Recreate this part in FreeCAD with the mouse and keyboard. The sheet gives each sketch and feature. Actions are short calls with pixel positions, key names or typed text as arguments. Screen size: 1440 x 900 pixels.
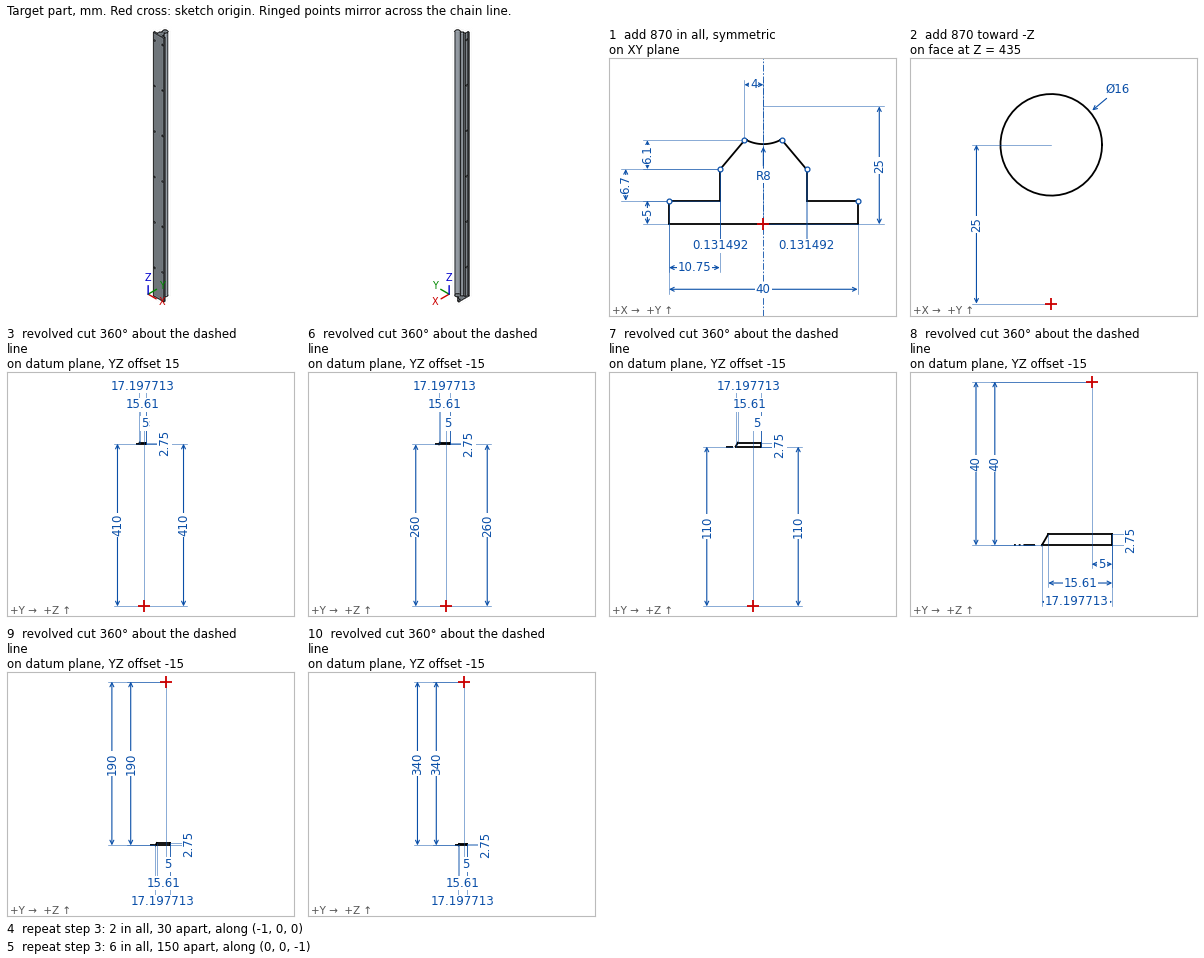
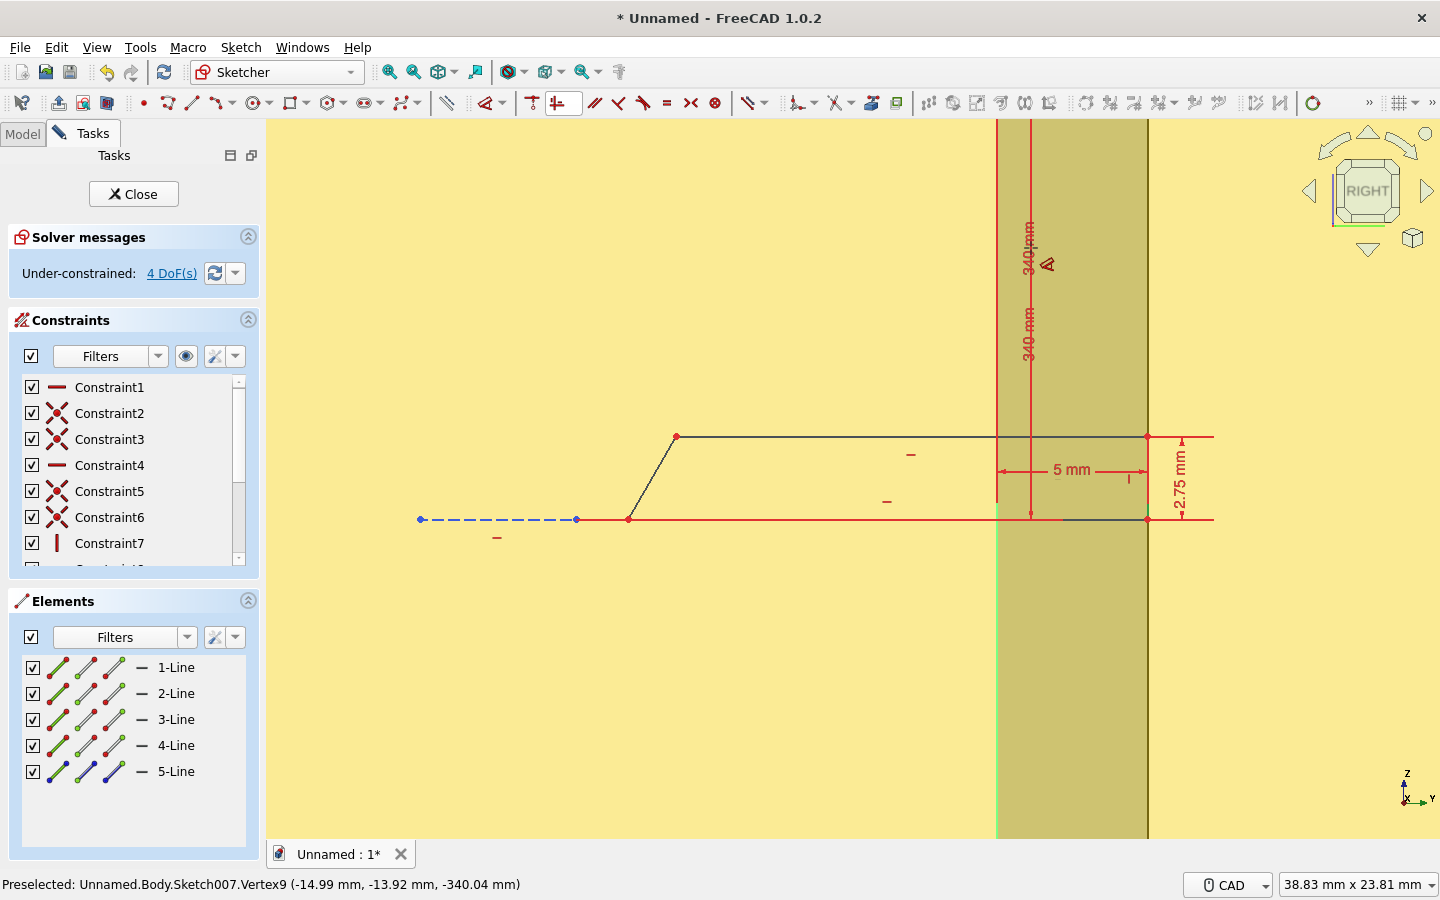
scroll(1006, 437, up, 2)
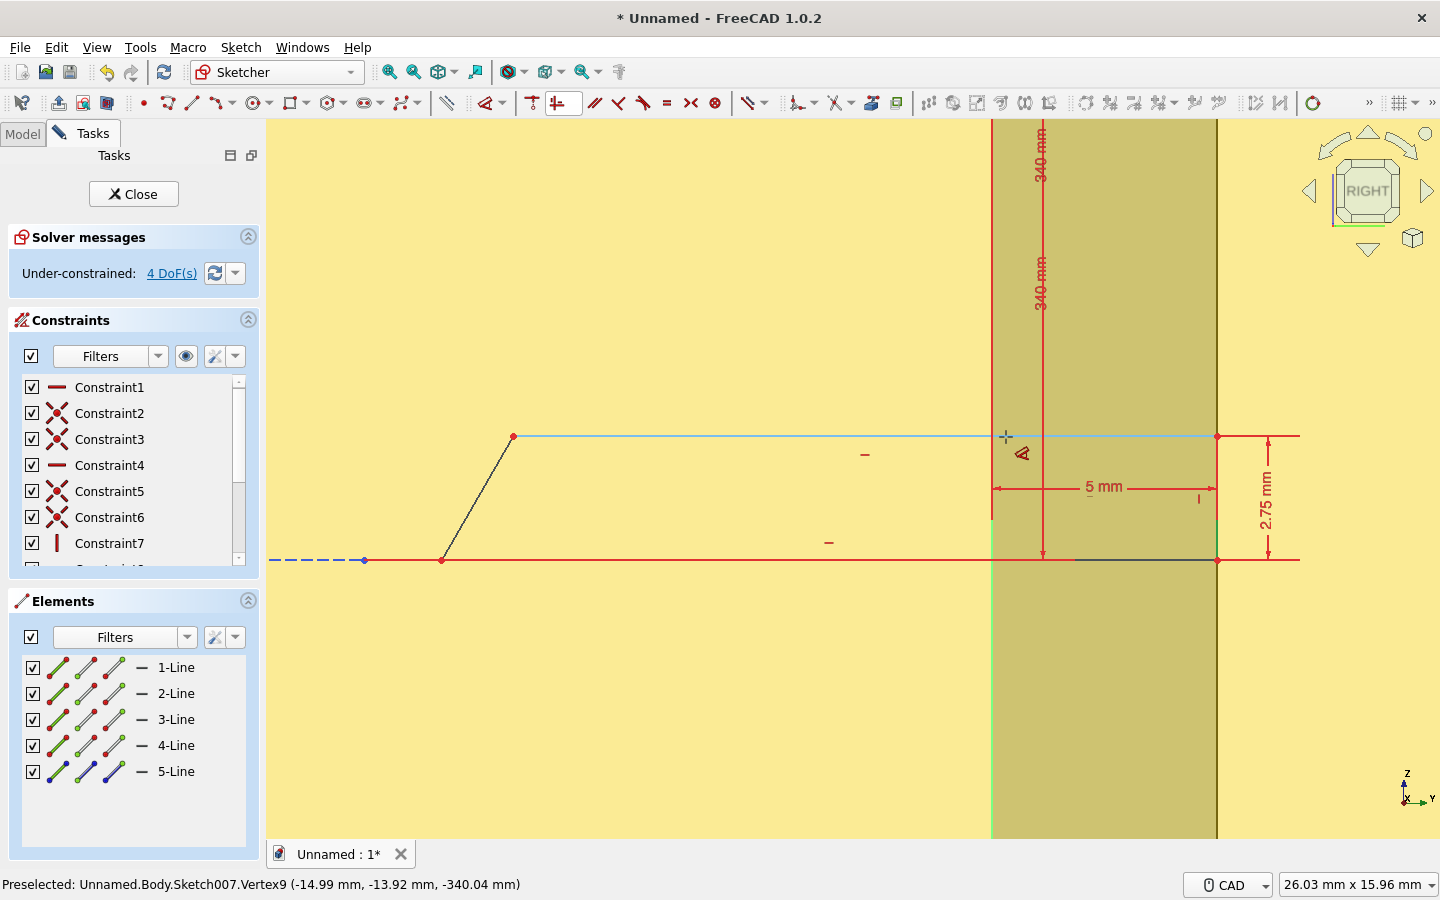
click(1006, 436)
click(865, 402)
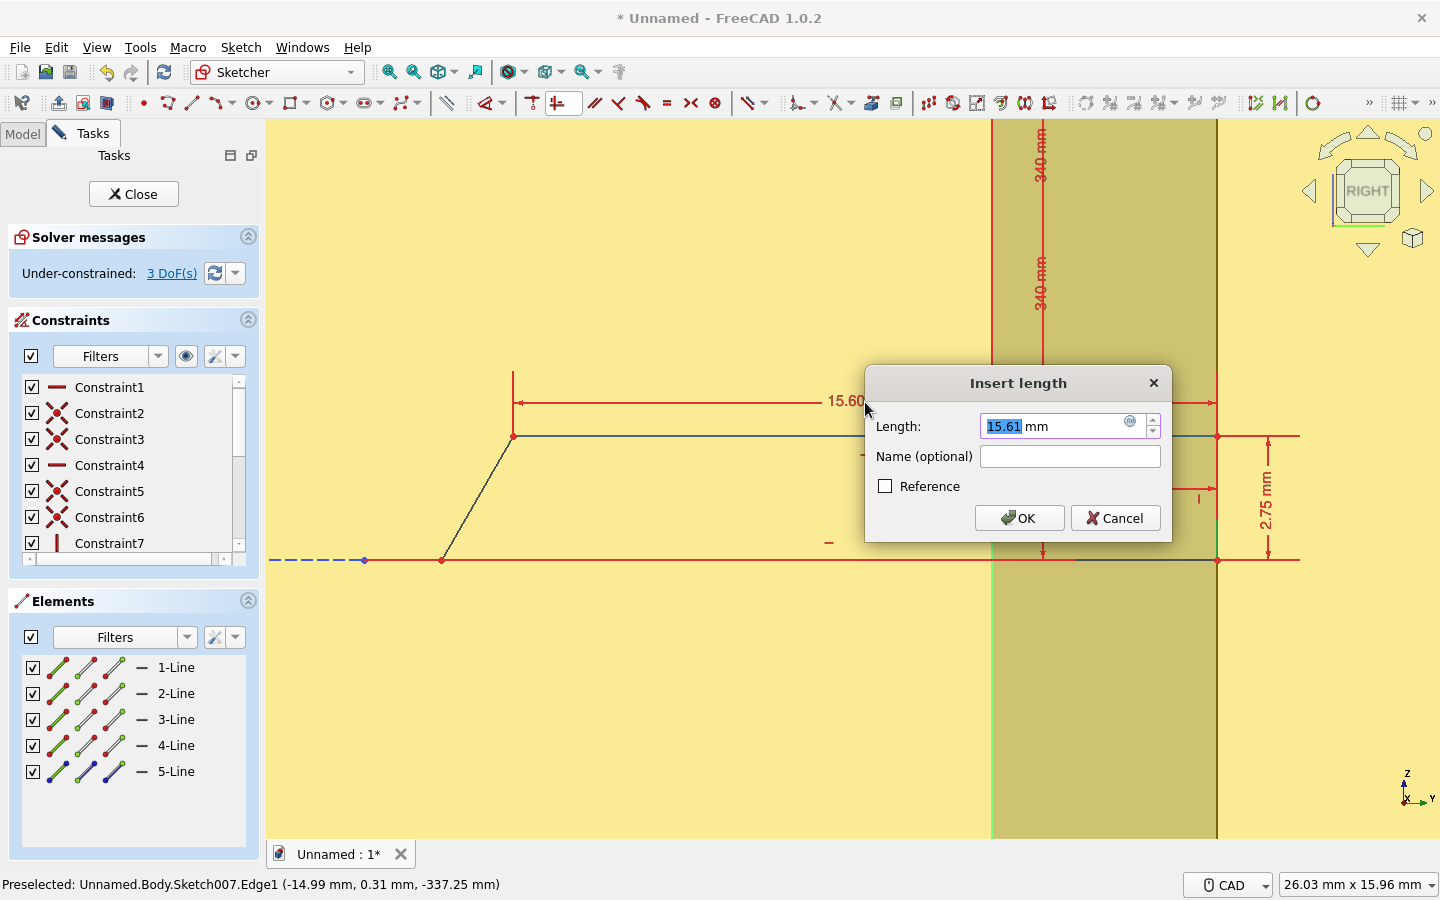
text(15.61)
key(Return)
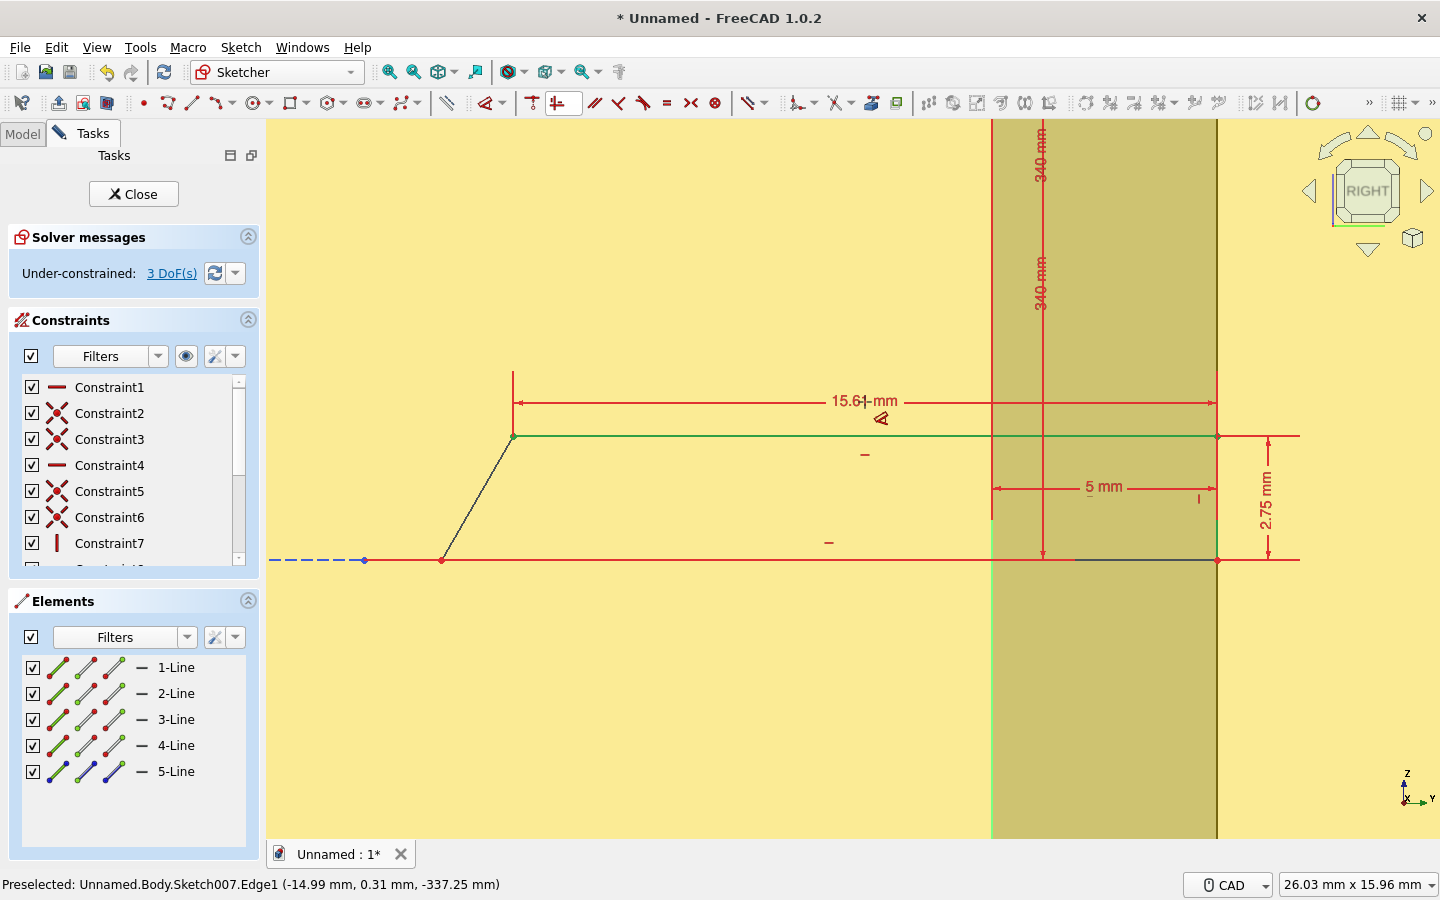
click(674, 560)
click(830, 594)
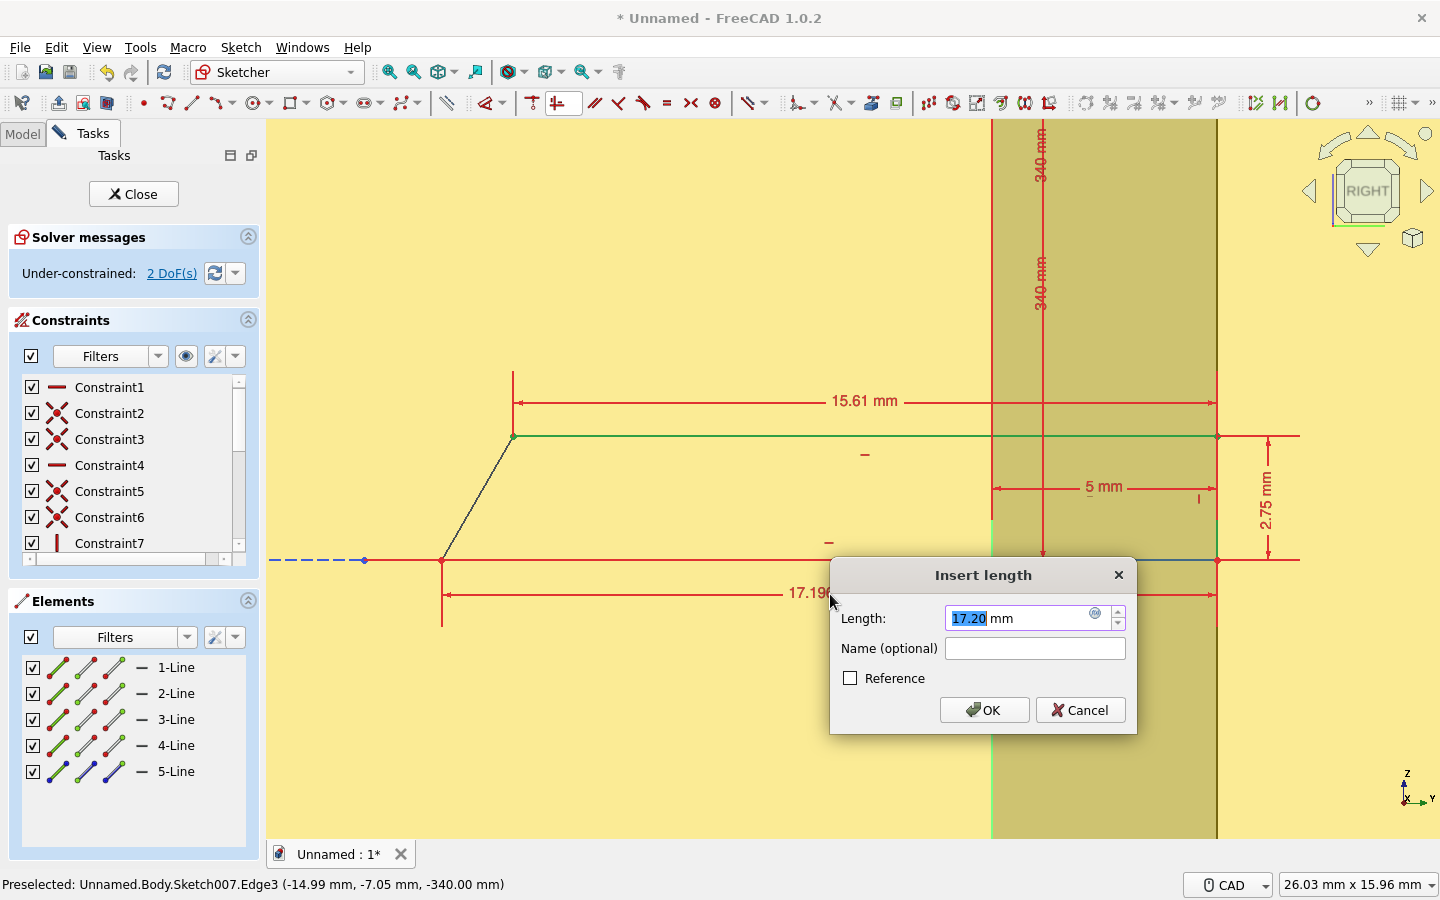
text(17.197713)
key(Return)
key(Escape)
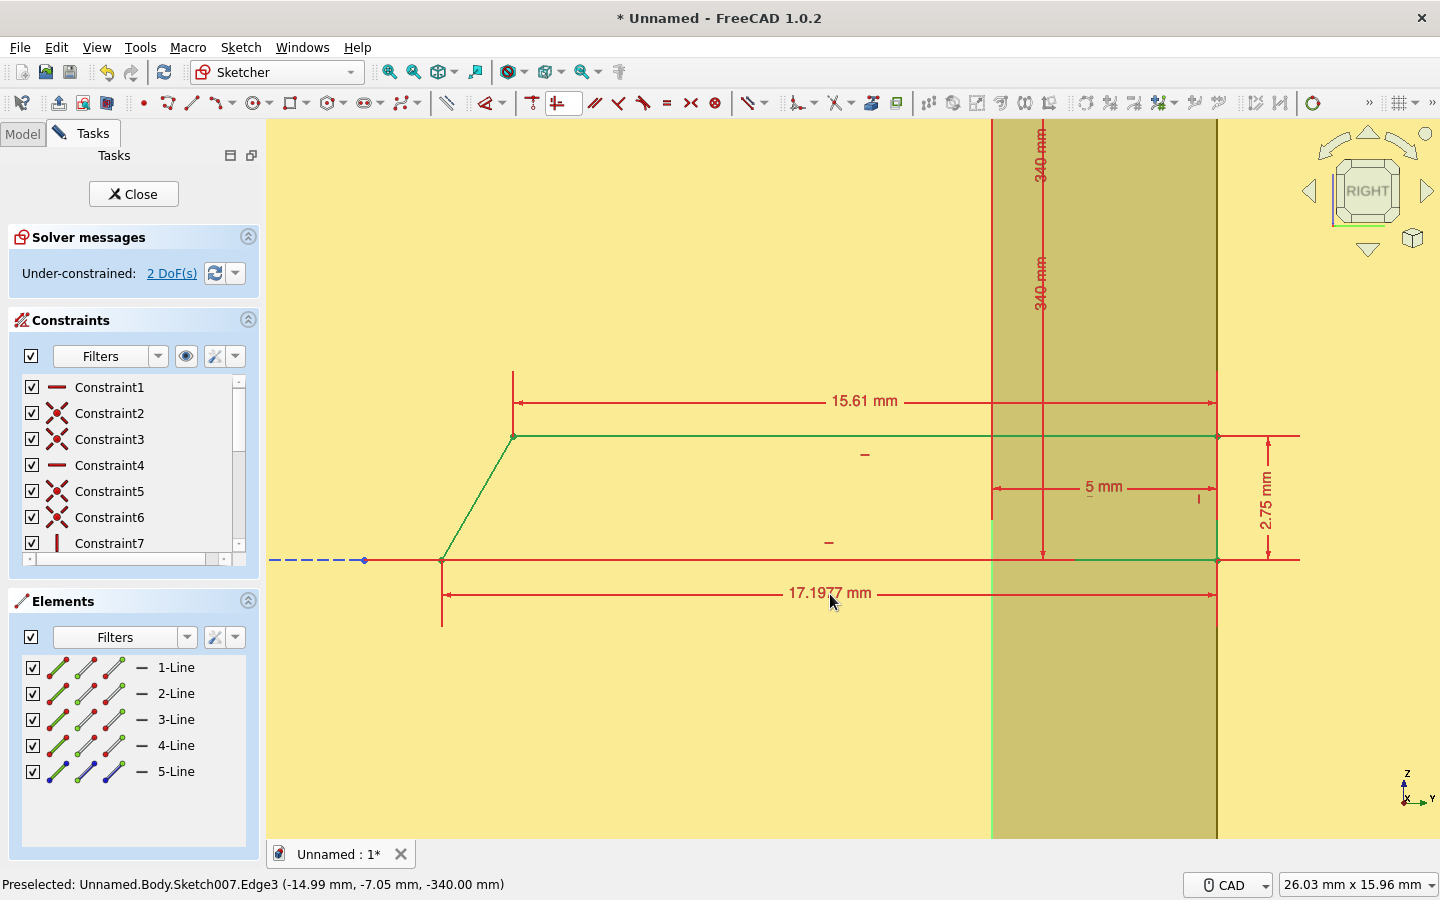
click(134, 194)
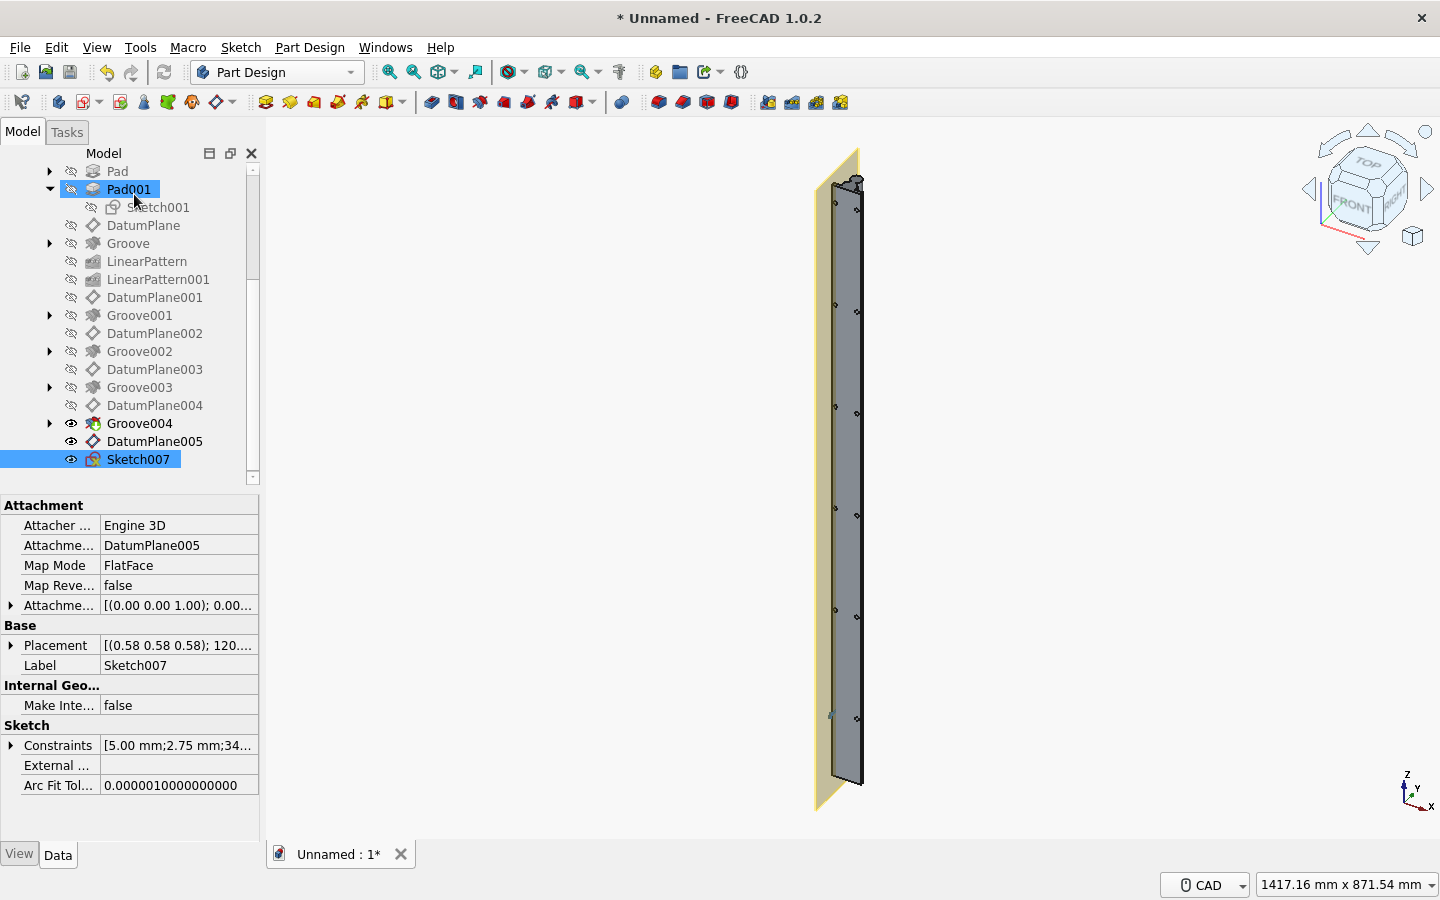
click(480, 102)